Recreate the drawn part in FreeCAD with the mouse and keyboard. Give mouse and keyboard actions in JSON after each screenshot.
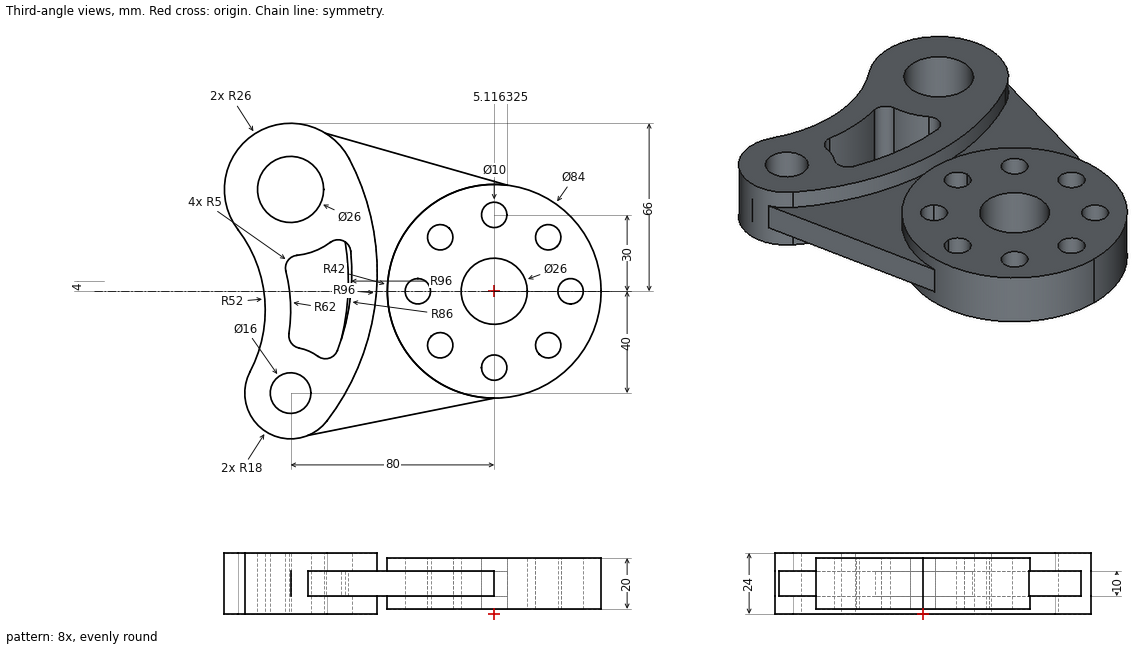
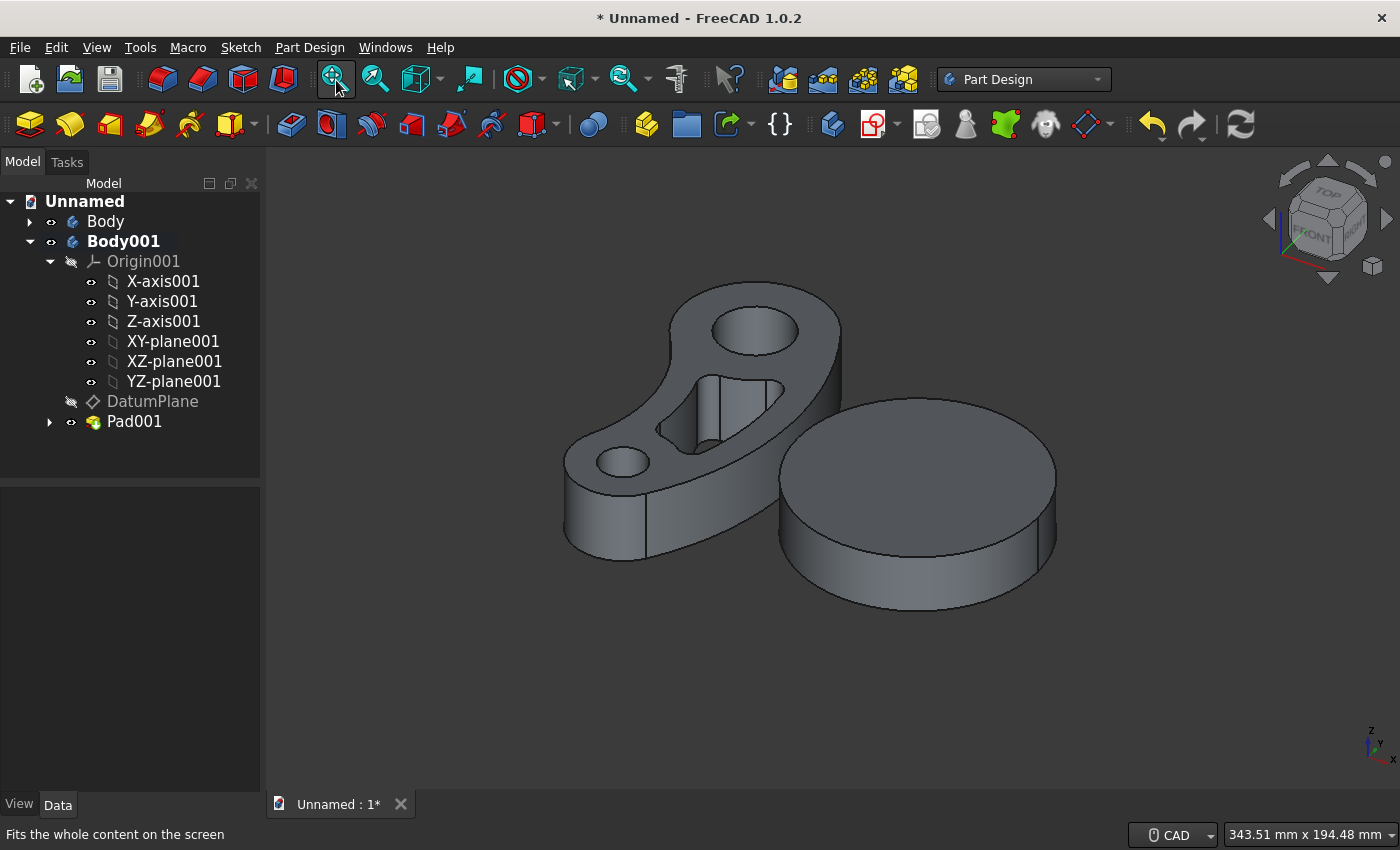
{"action": "double_click", "coordinate": [96, 222]}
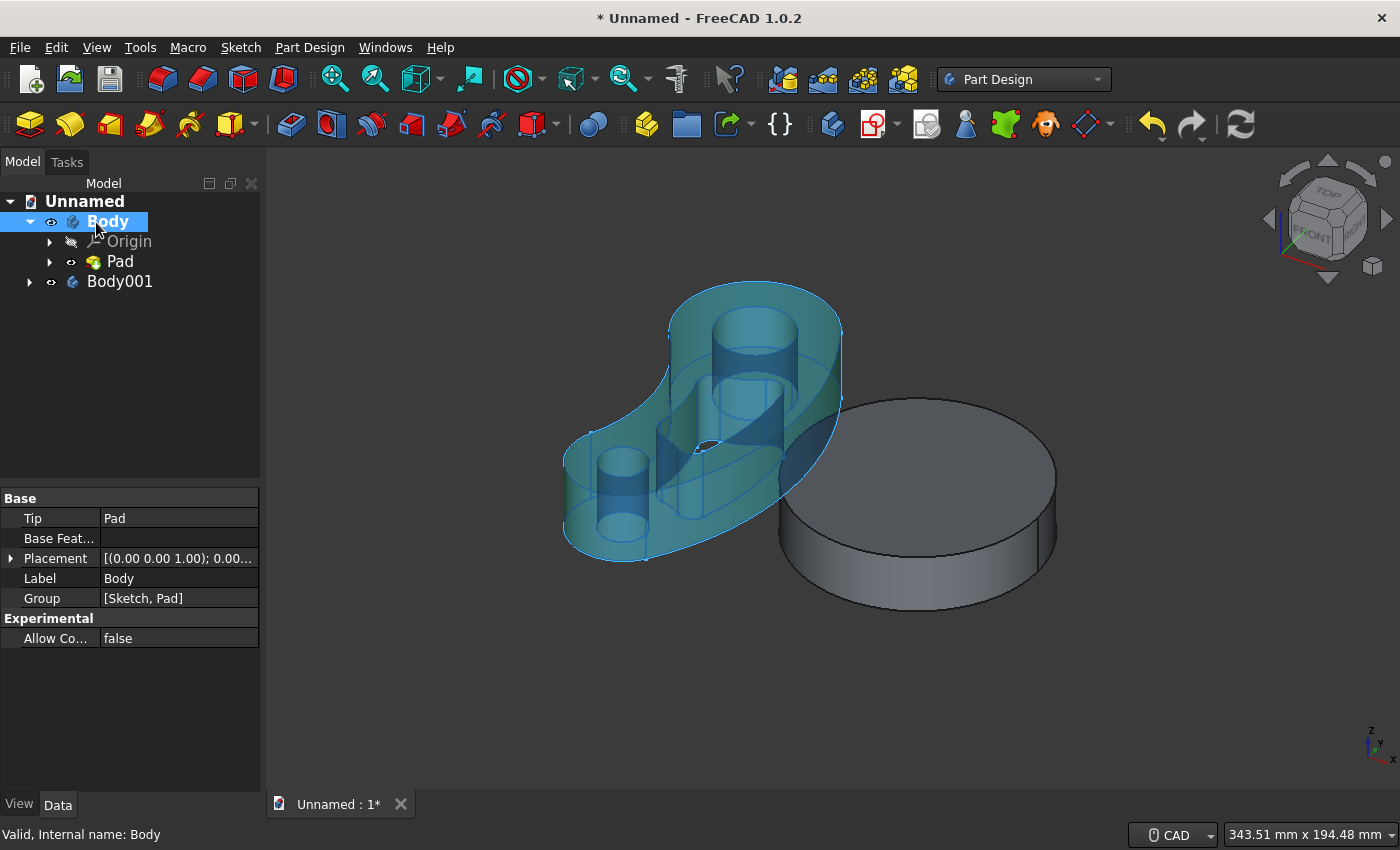
{"action": "left_click", "coordinate": [96, 222]}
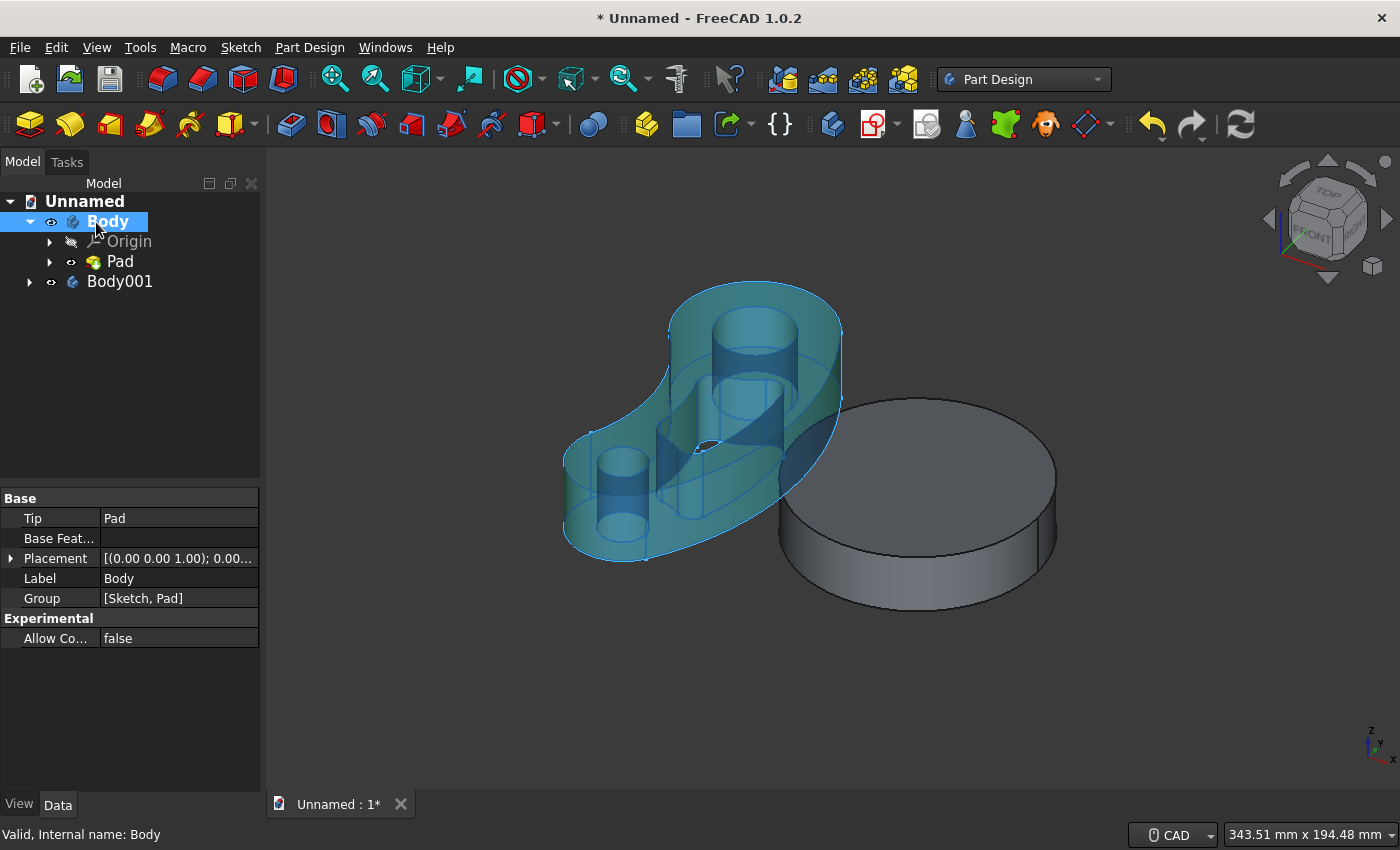
{"action": "left_click", "coordinate": [146, 638]}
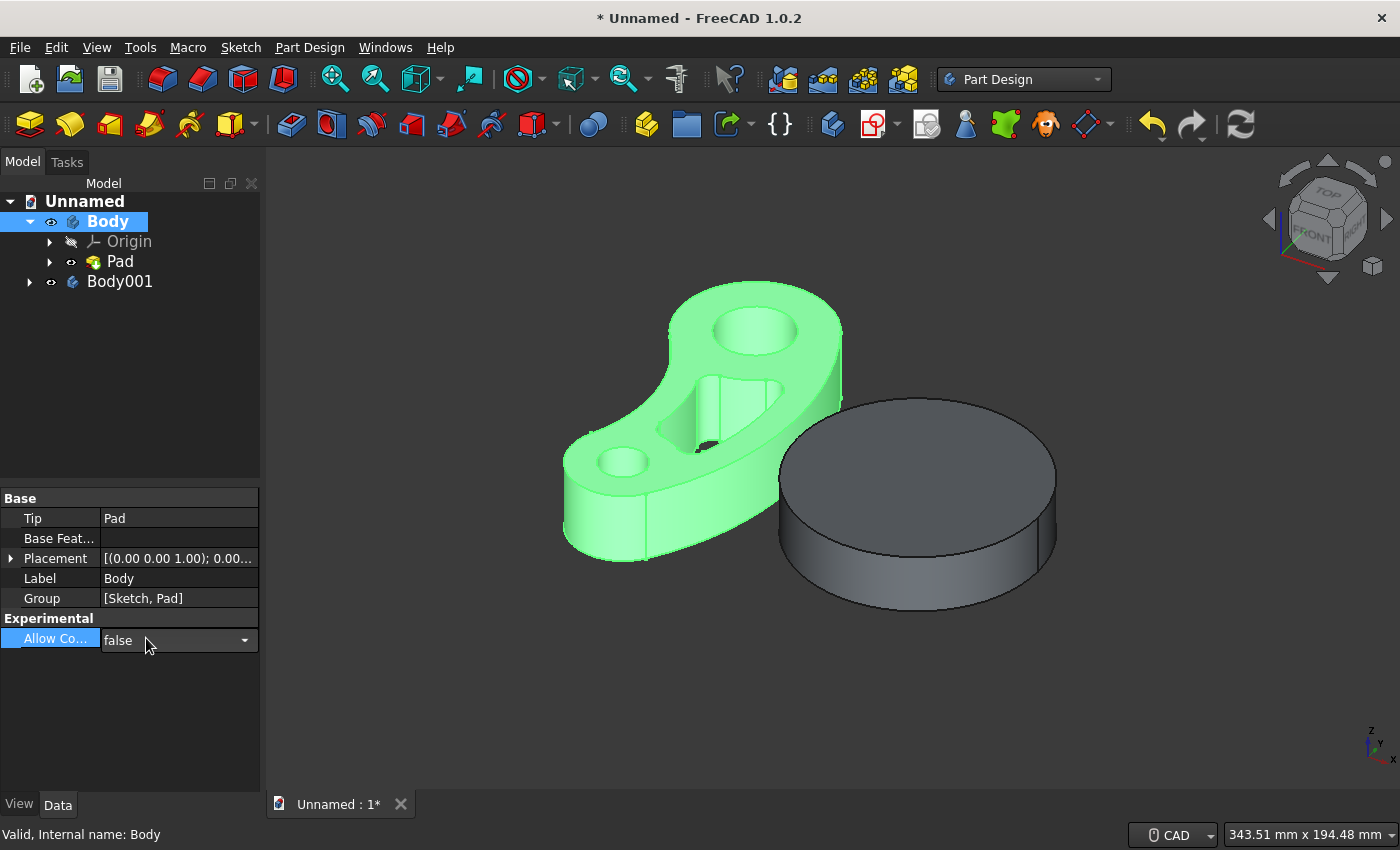
{"action": "left_click", "coordinate": [146, 638]}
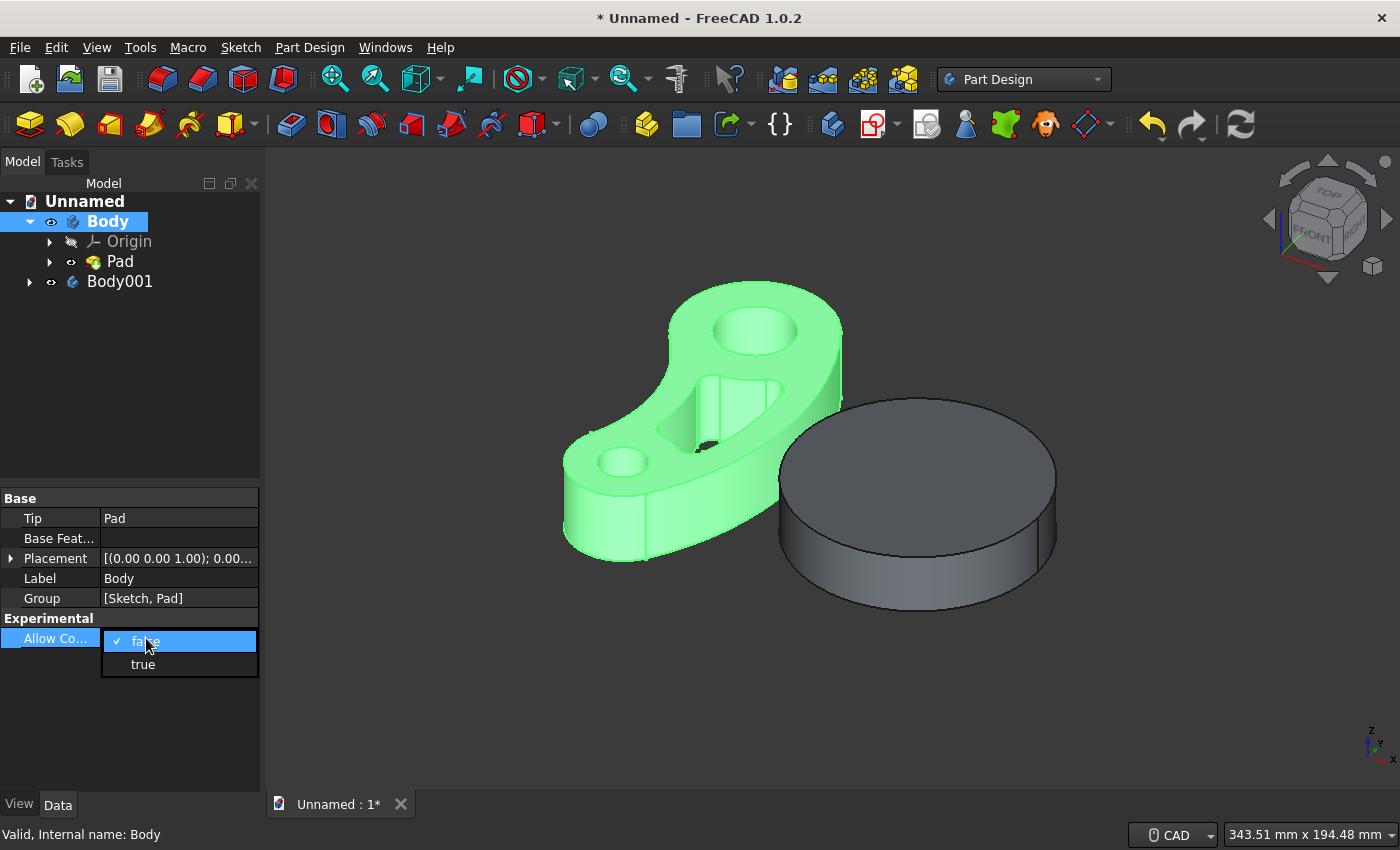
{"action": "left_click", "coordinate": [179, 664]}
{"action": "key", "text": "Return"}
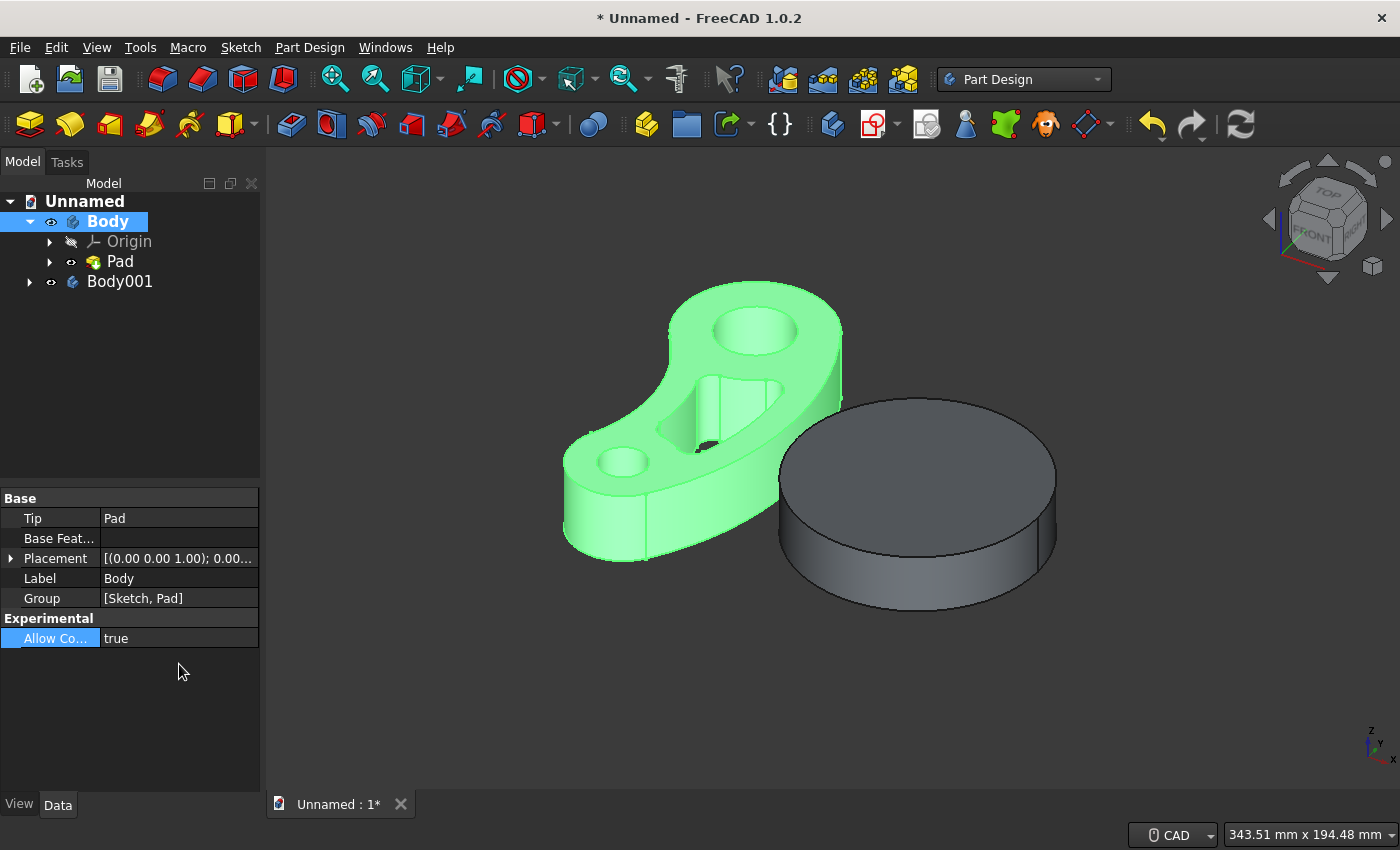
{"action": "left_click", "coordinate": [96, 282]}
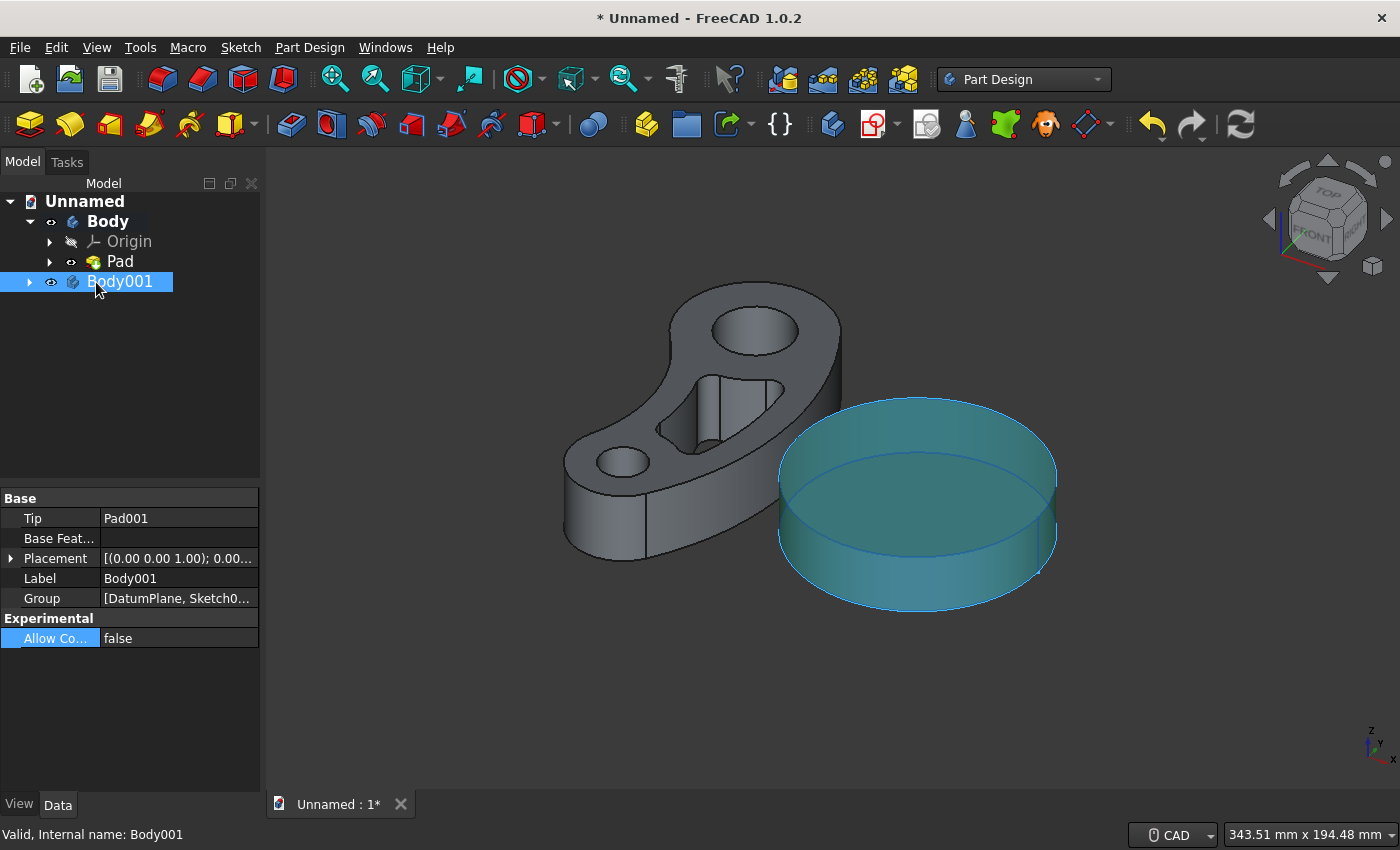
{"action": "left_click", "coordinate": [594, 124]}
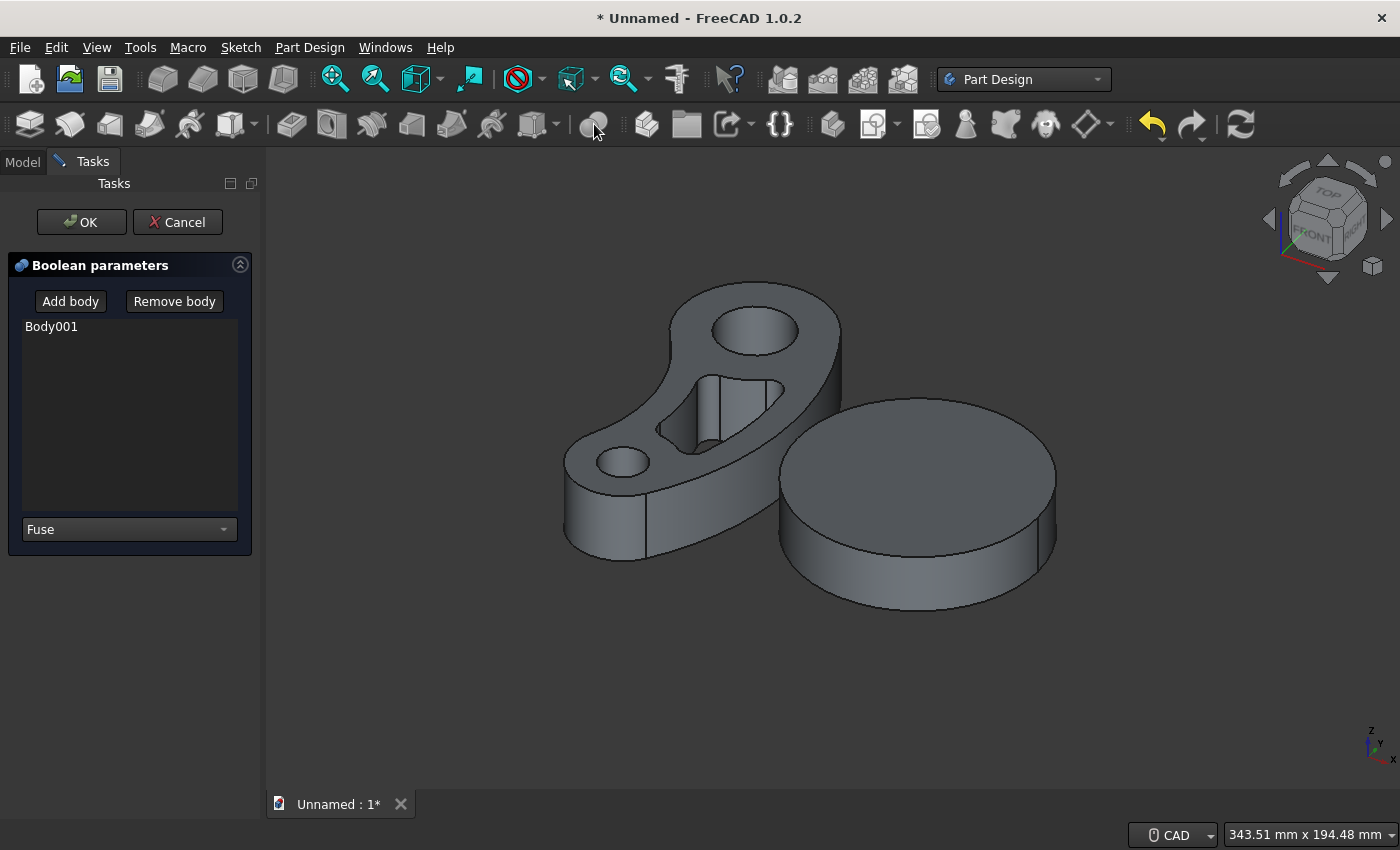
{"action": "left_click", "coordinate": [82, 222]}